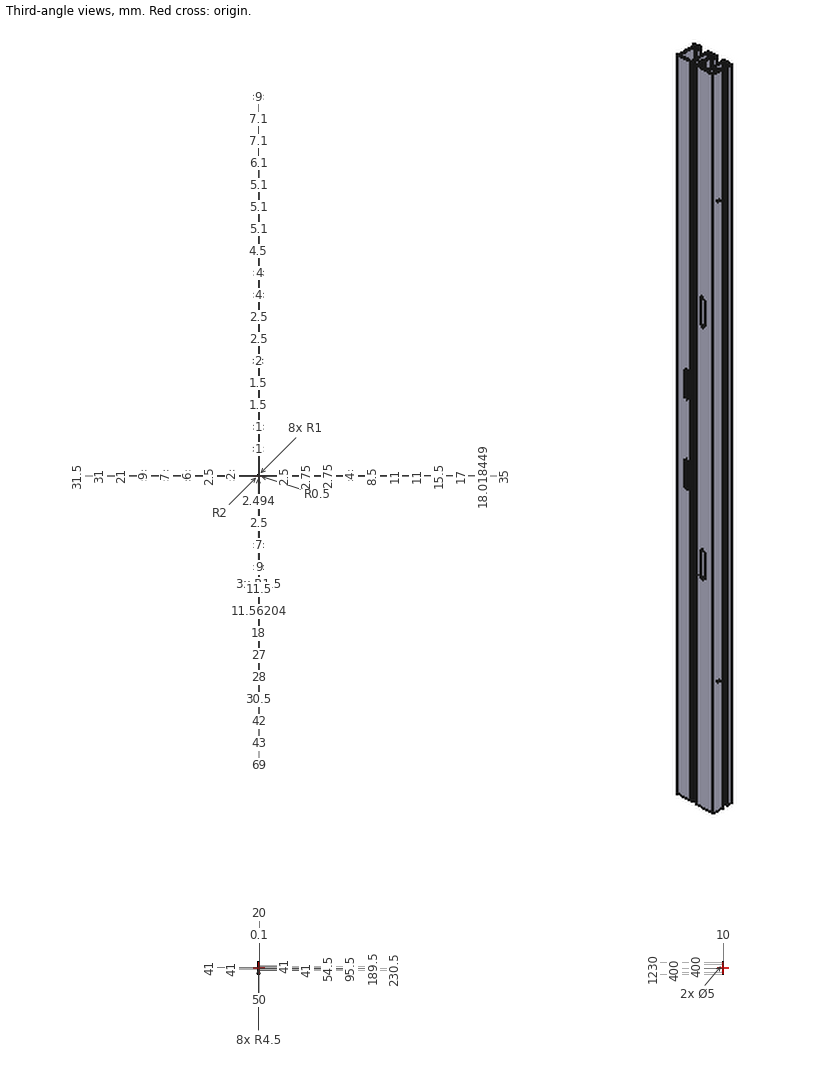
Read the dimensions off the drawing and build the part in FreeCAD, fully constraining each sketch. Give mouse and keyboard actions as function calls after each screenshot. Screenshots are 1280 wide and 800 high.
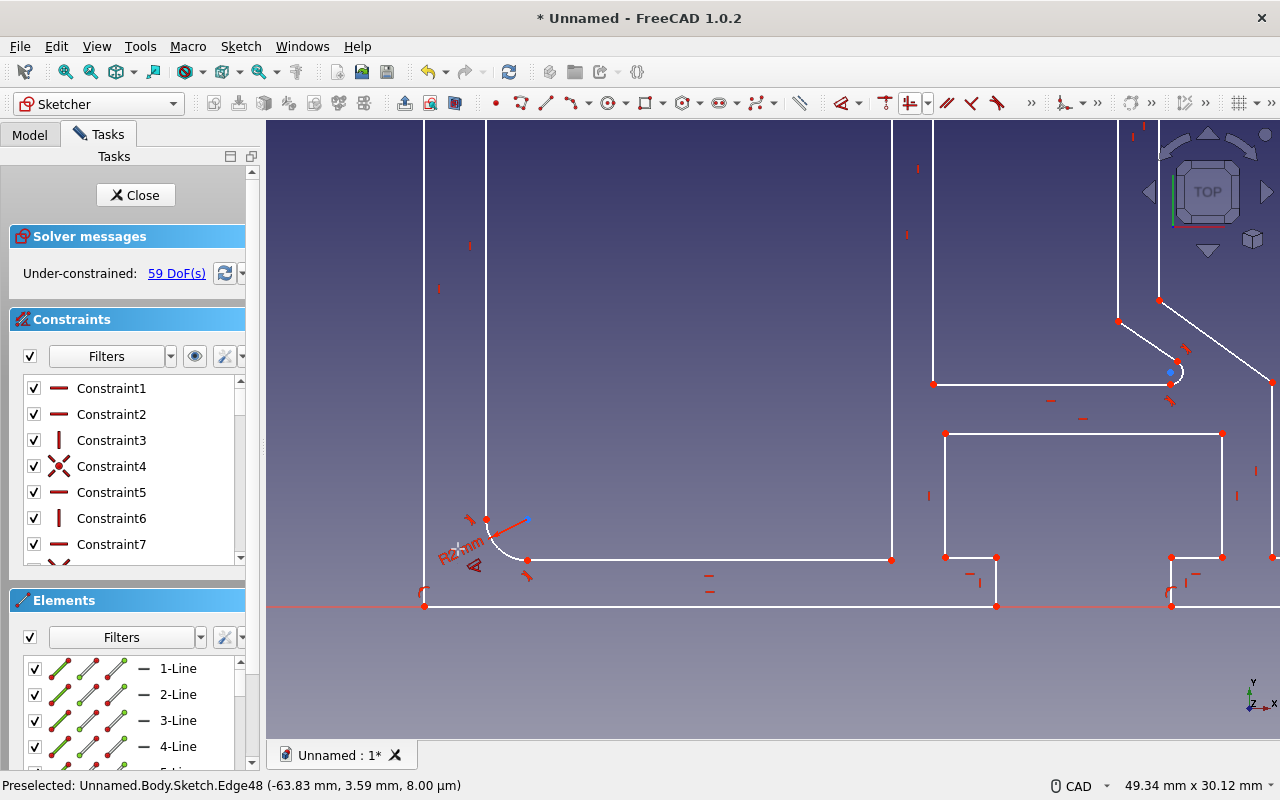
scroll(487, 536, down, 5)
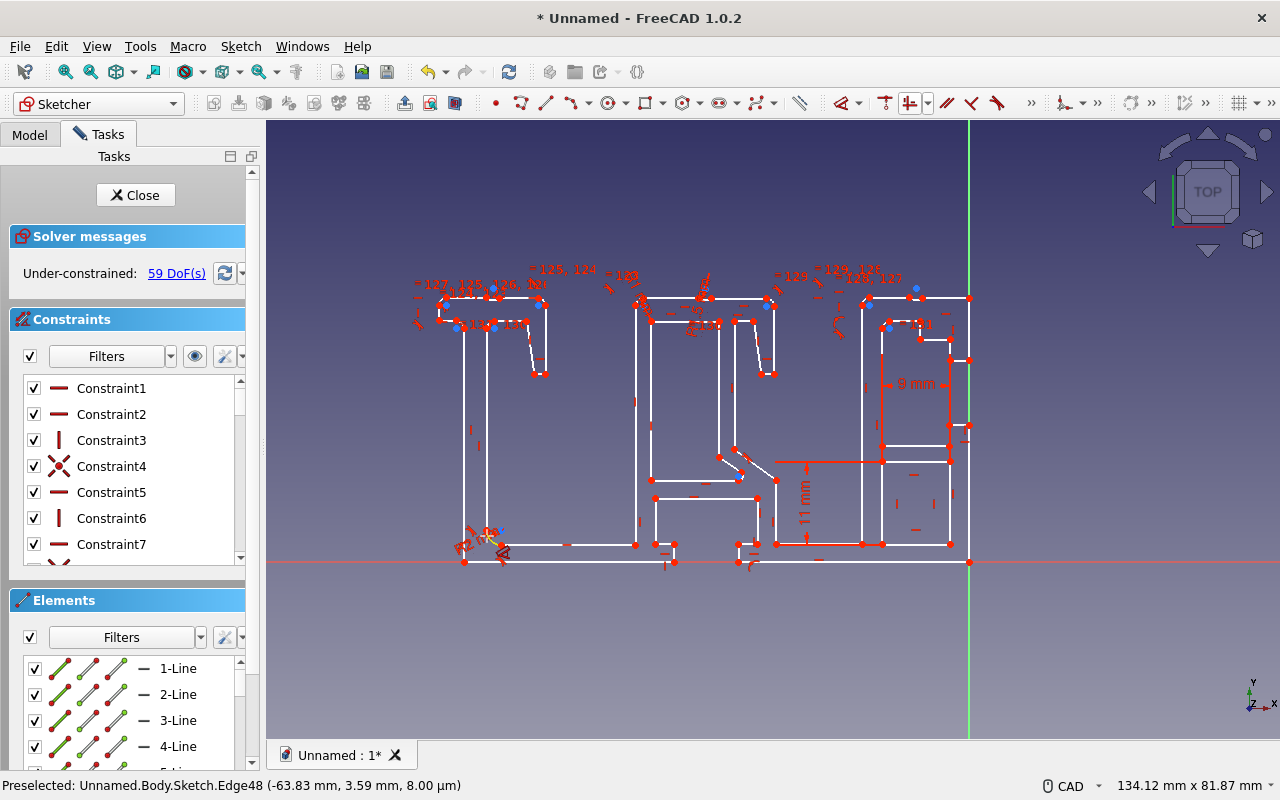
scroll(742, 479, up, 12)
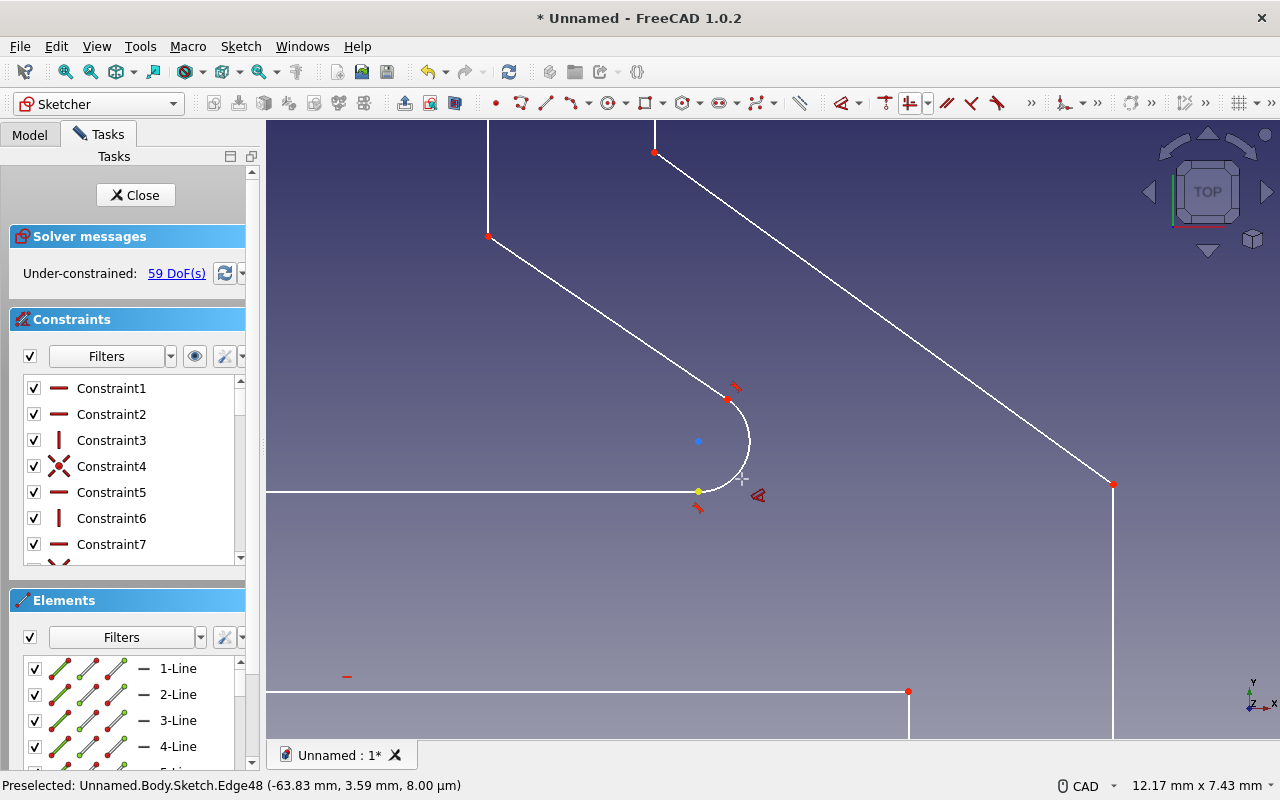
click(734, 478)
click(756, 501)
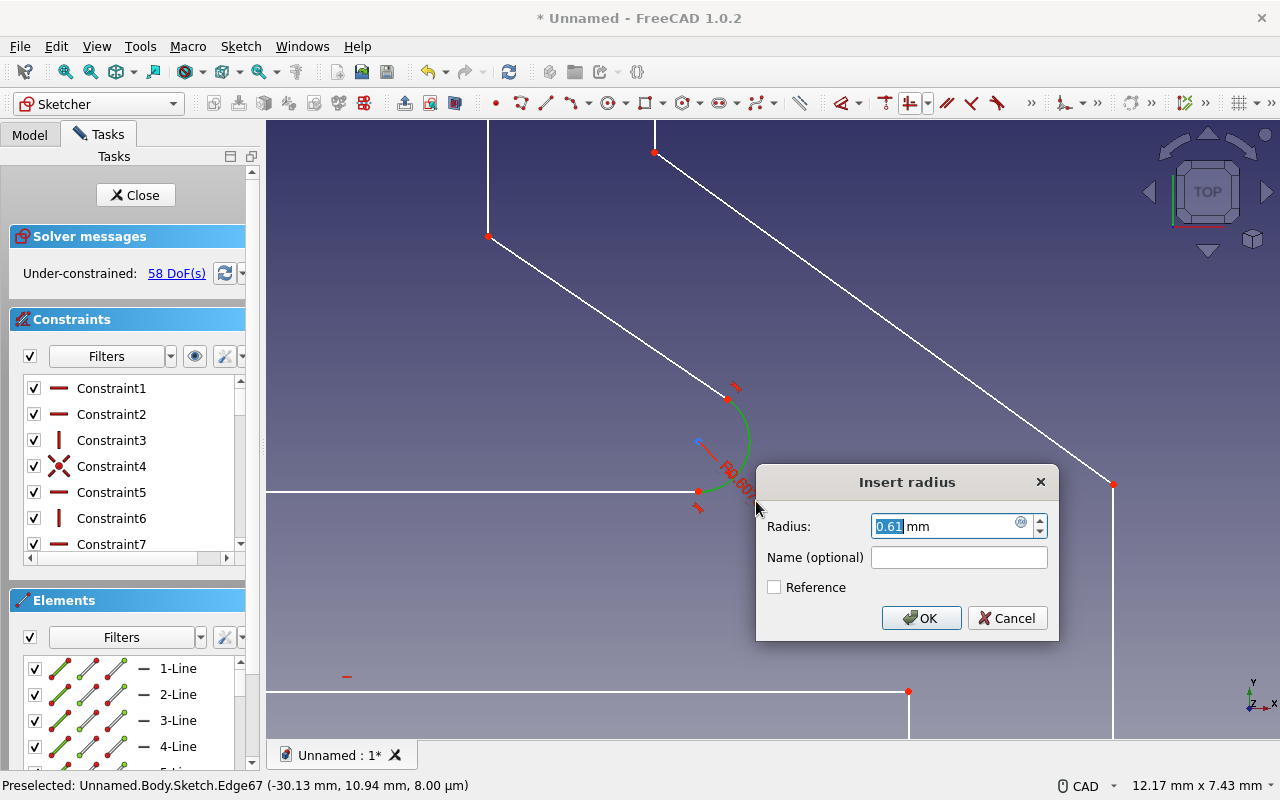
text(0.5)
key(Return)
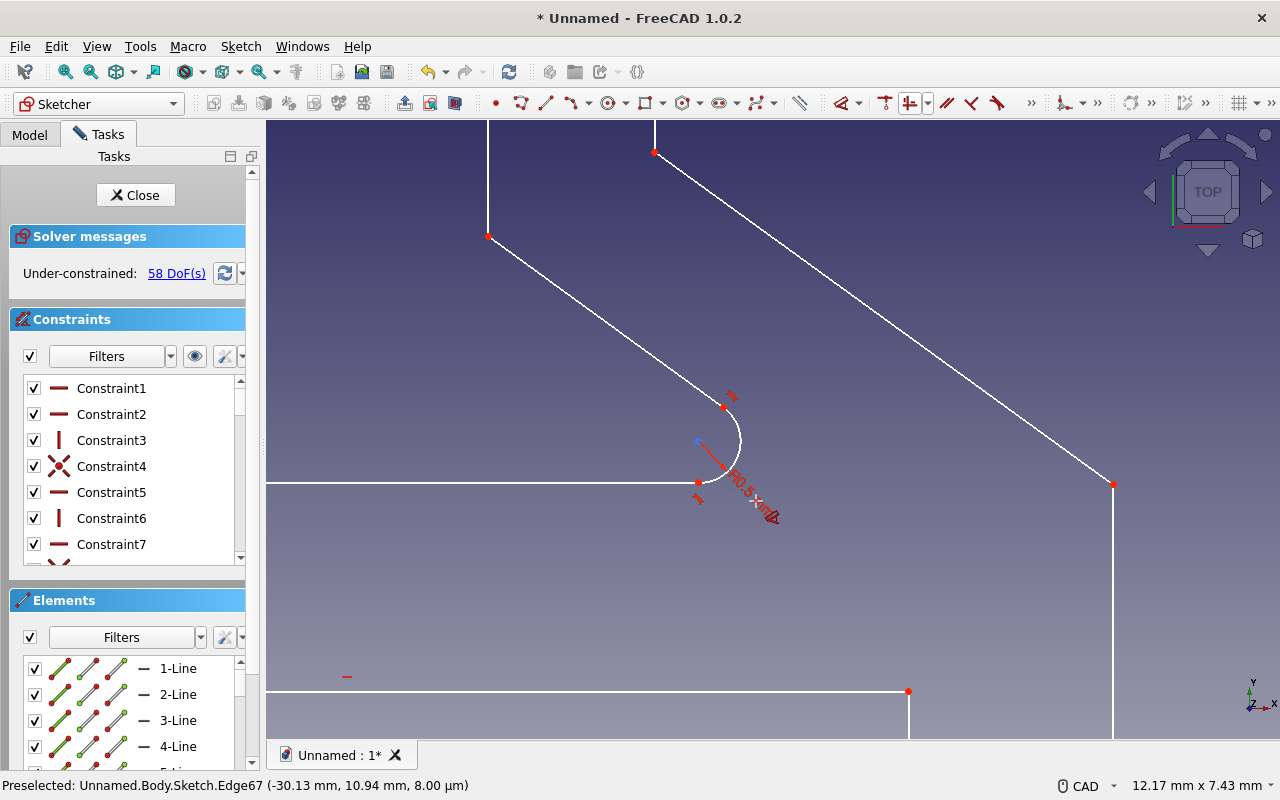
scroll(742, 479, down, 12)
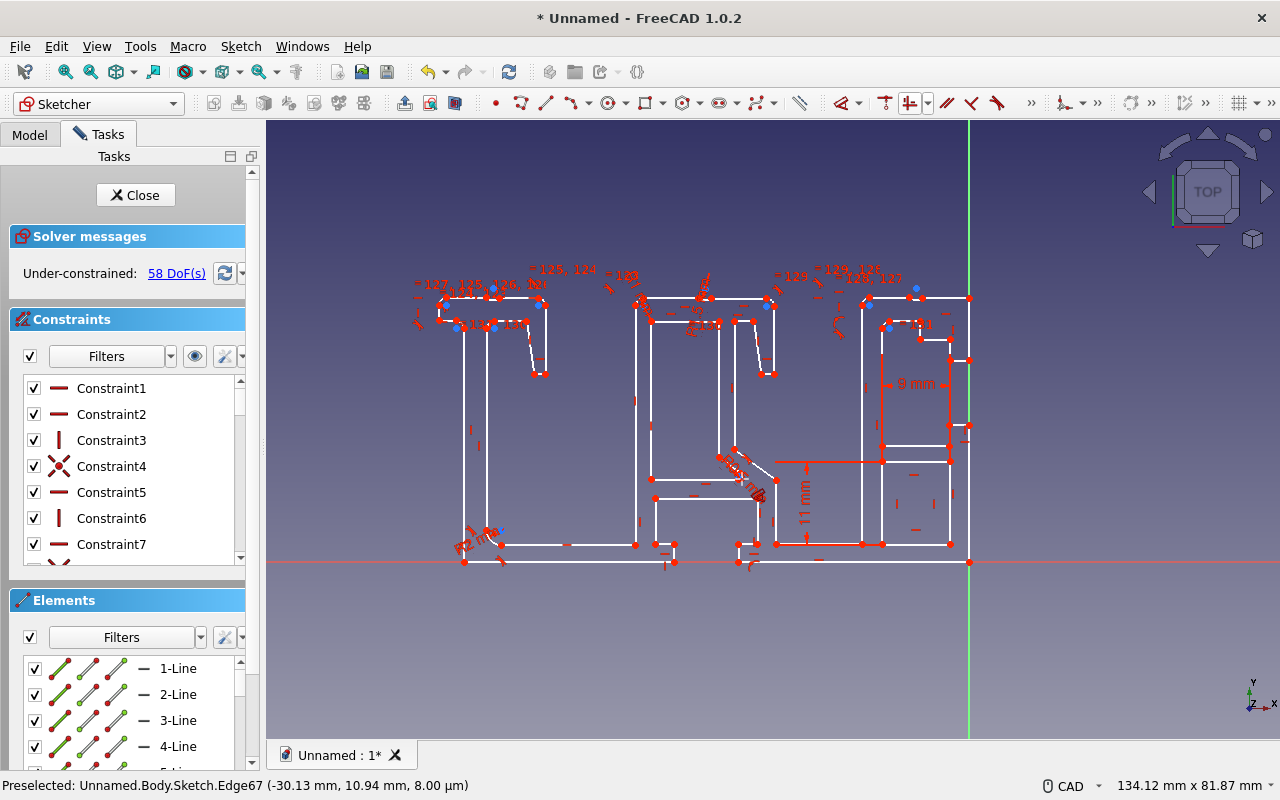
click(546, 354)
click(512, 340)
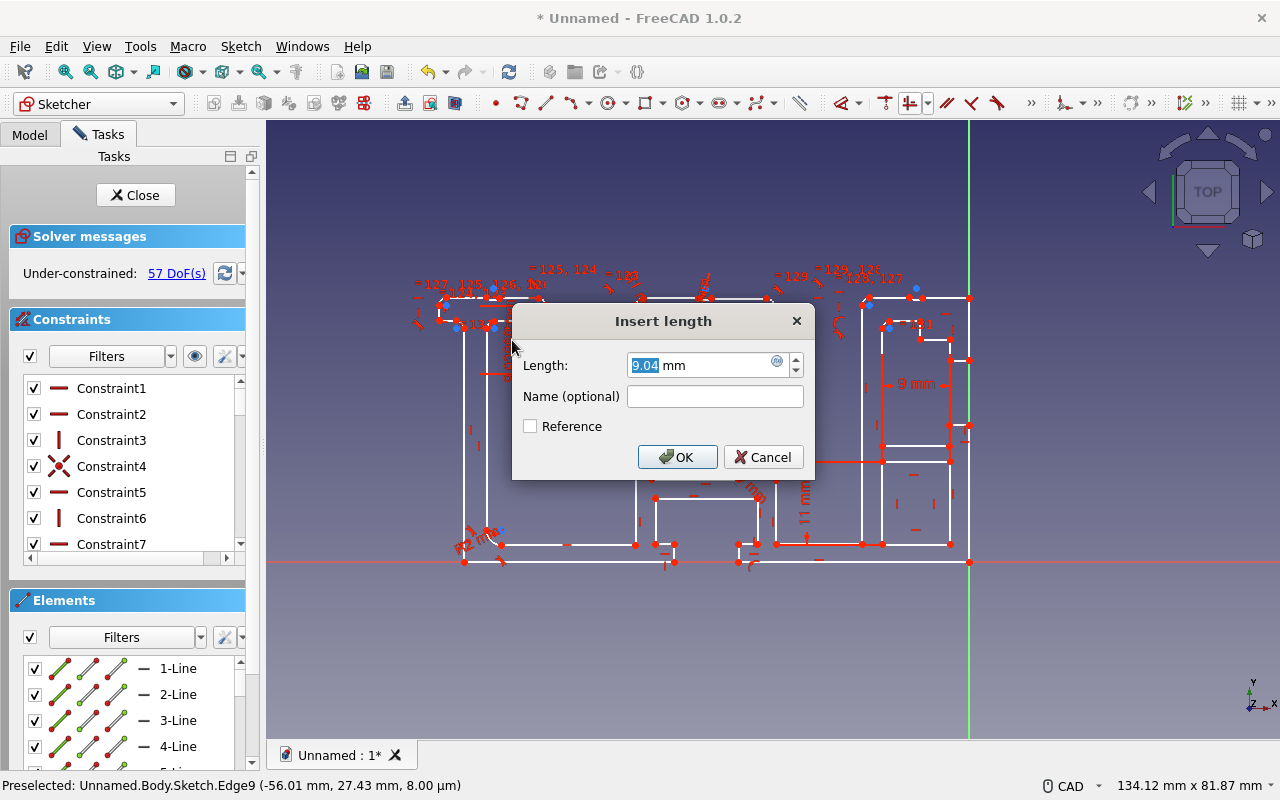
text(9)
key(Return)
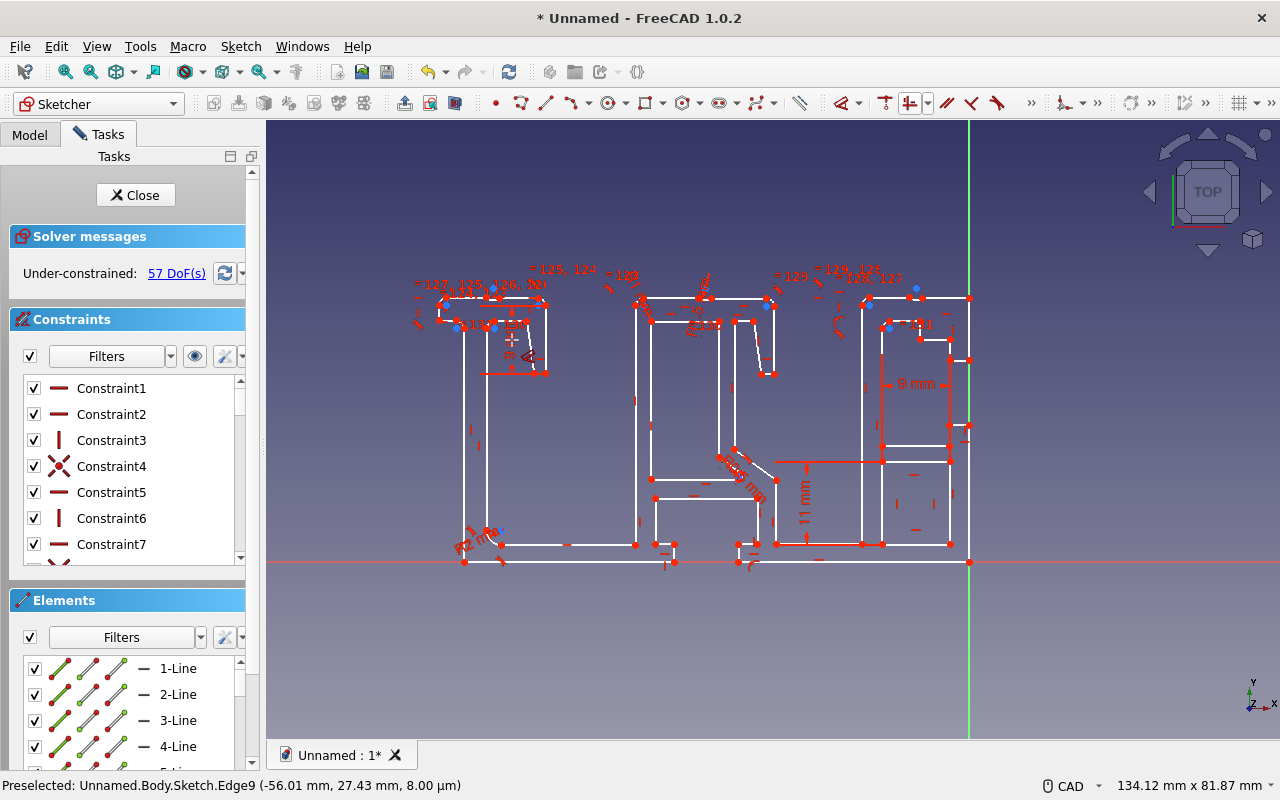
scroll(439, 313, up, 5)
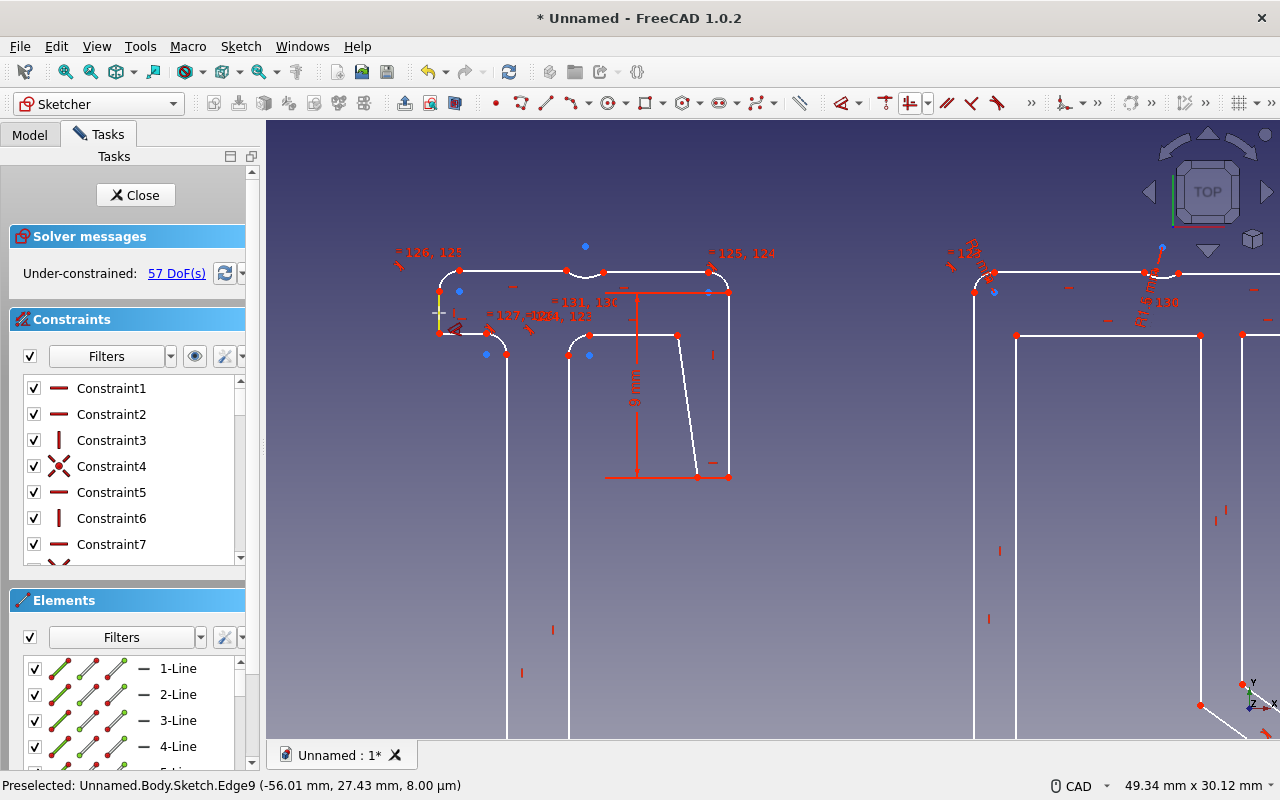
click(439, 313)
click(405, 313)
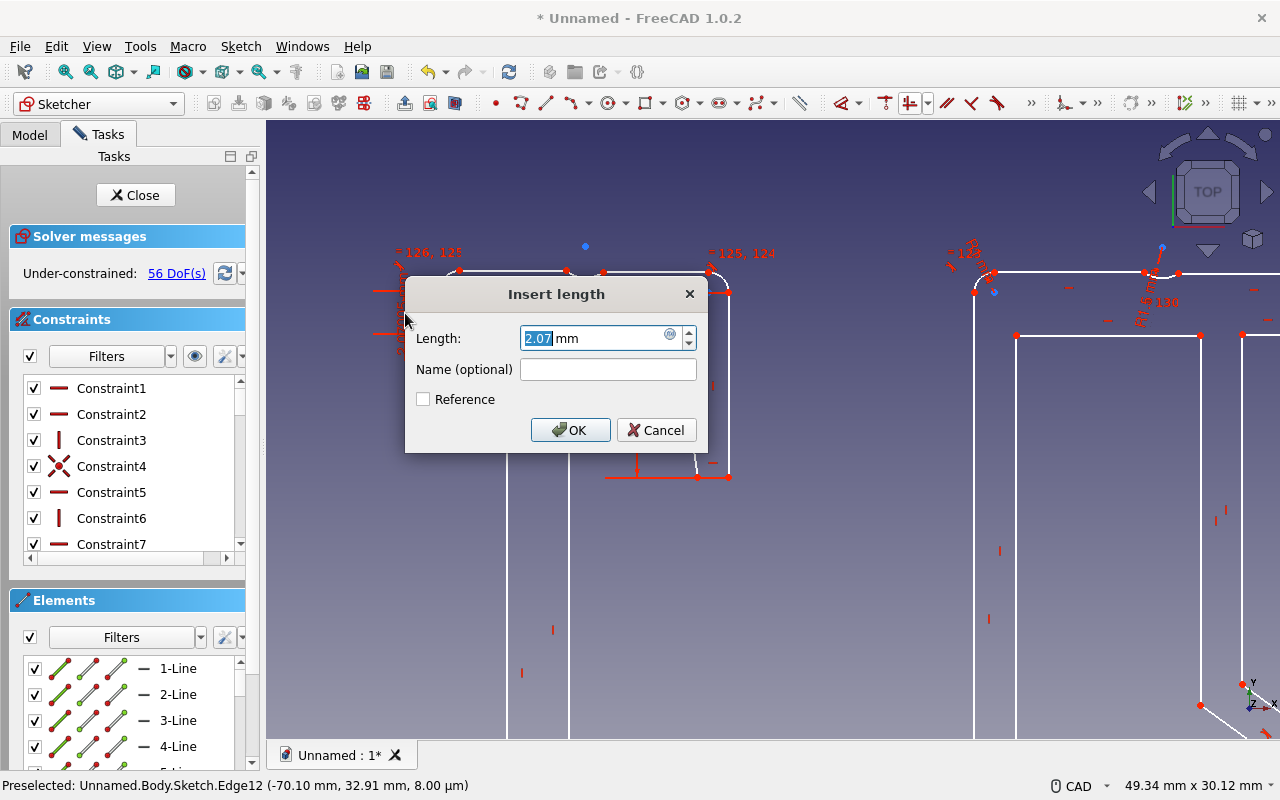
text(2)
key(Return)